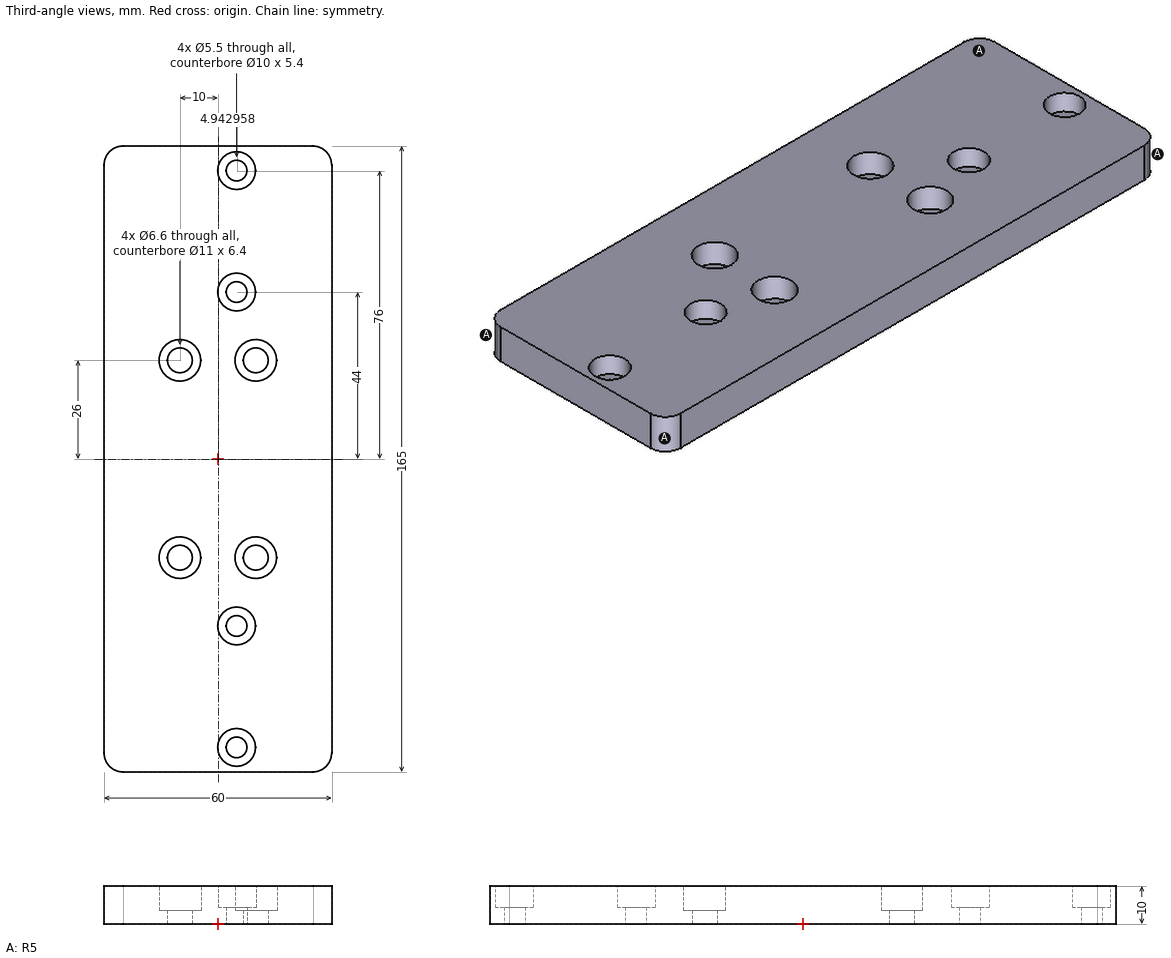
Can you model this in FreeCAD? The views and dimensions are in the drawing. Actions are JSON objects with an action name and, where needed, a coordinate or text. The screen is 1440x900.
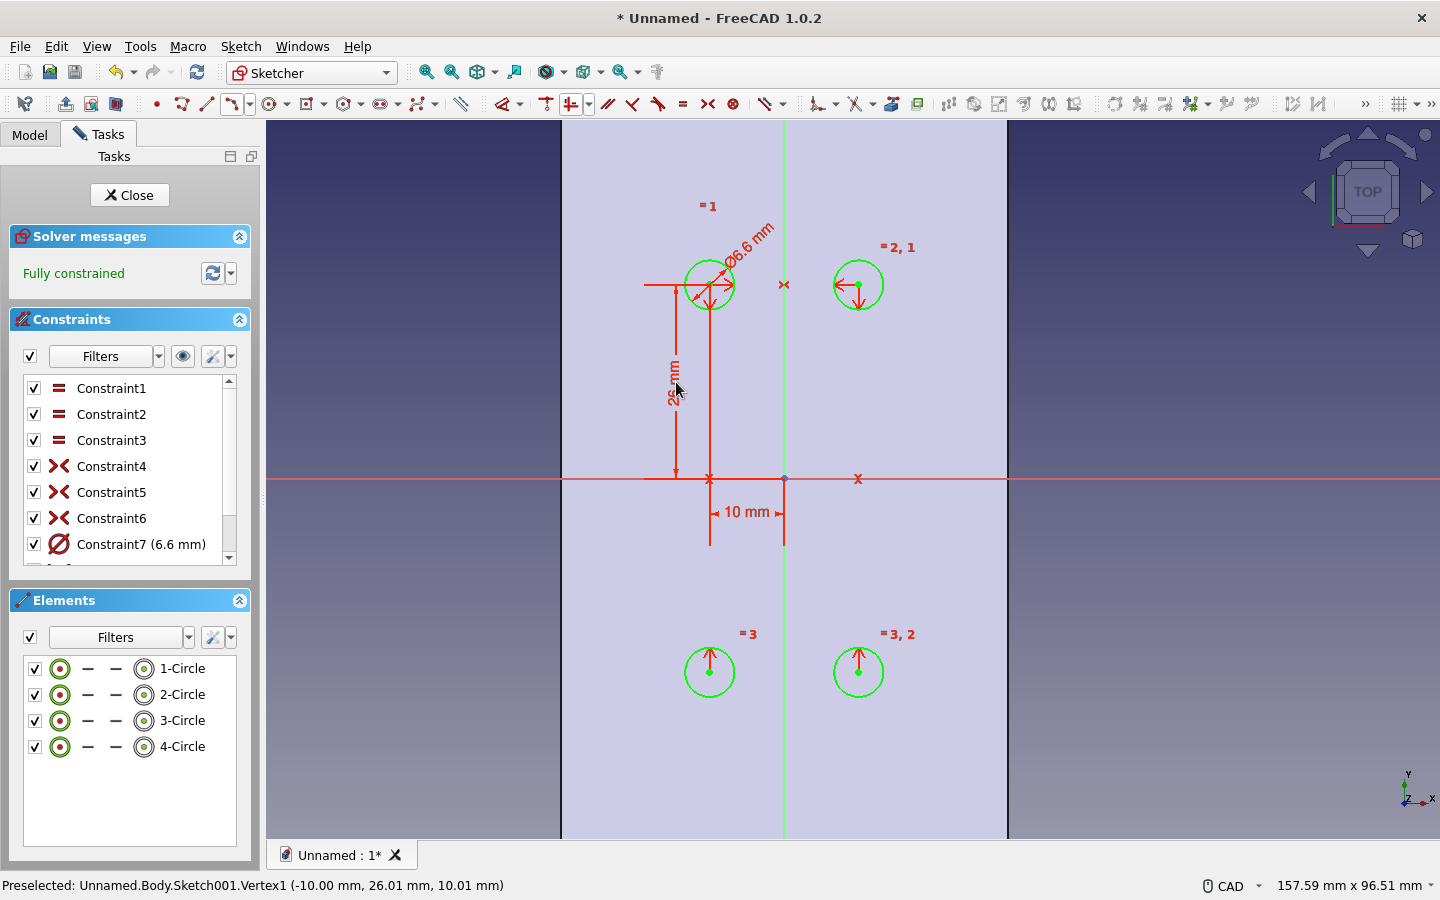
{"action": "left_click", "coordinate": [130, 195]}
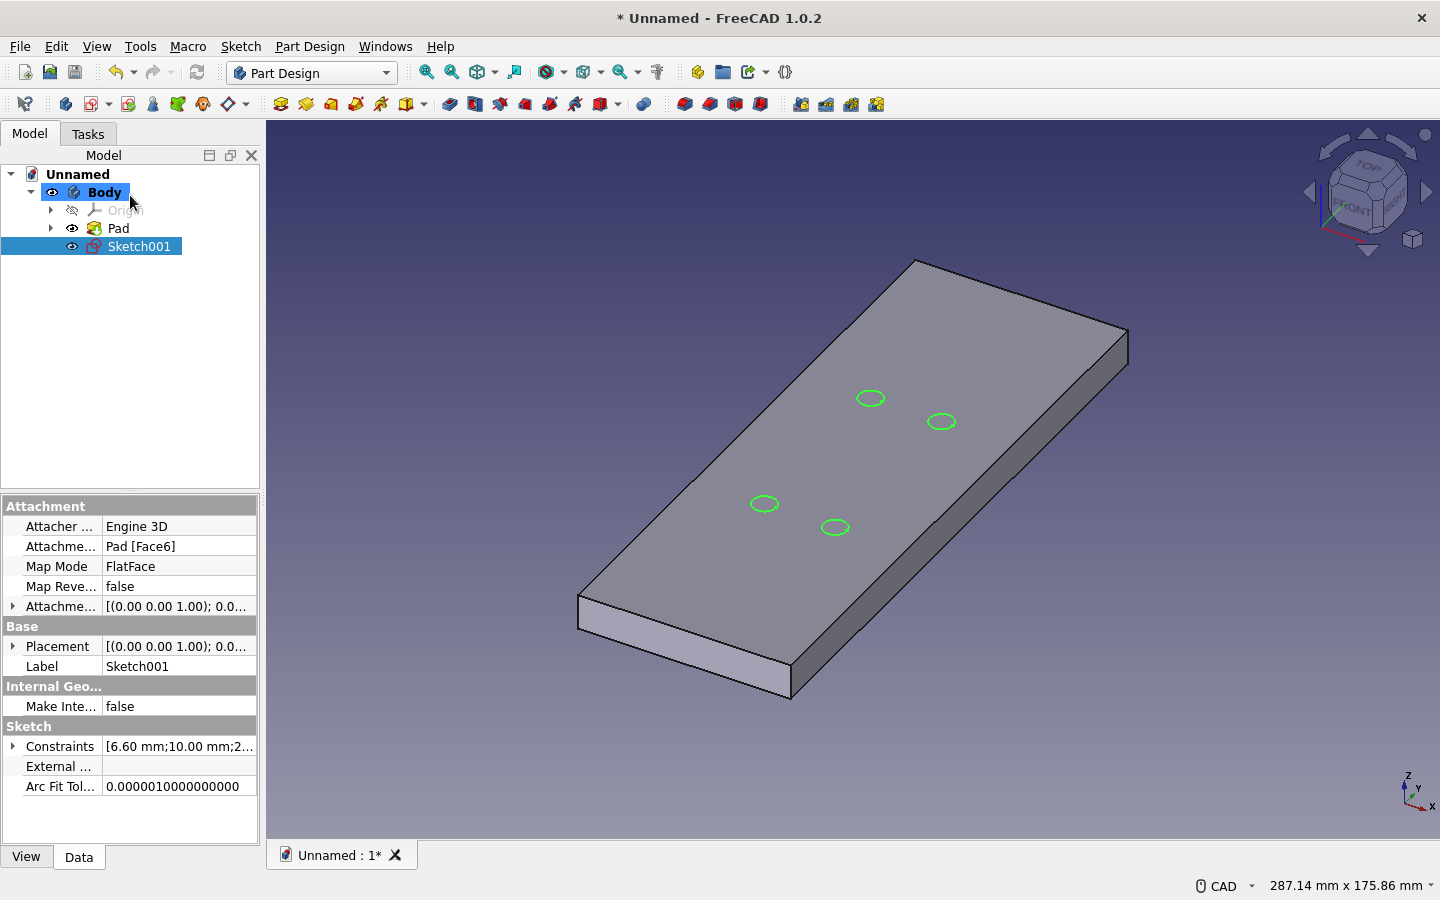
{"action": "left_click", "coordinate": [475, 104]}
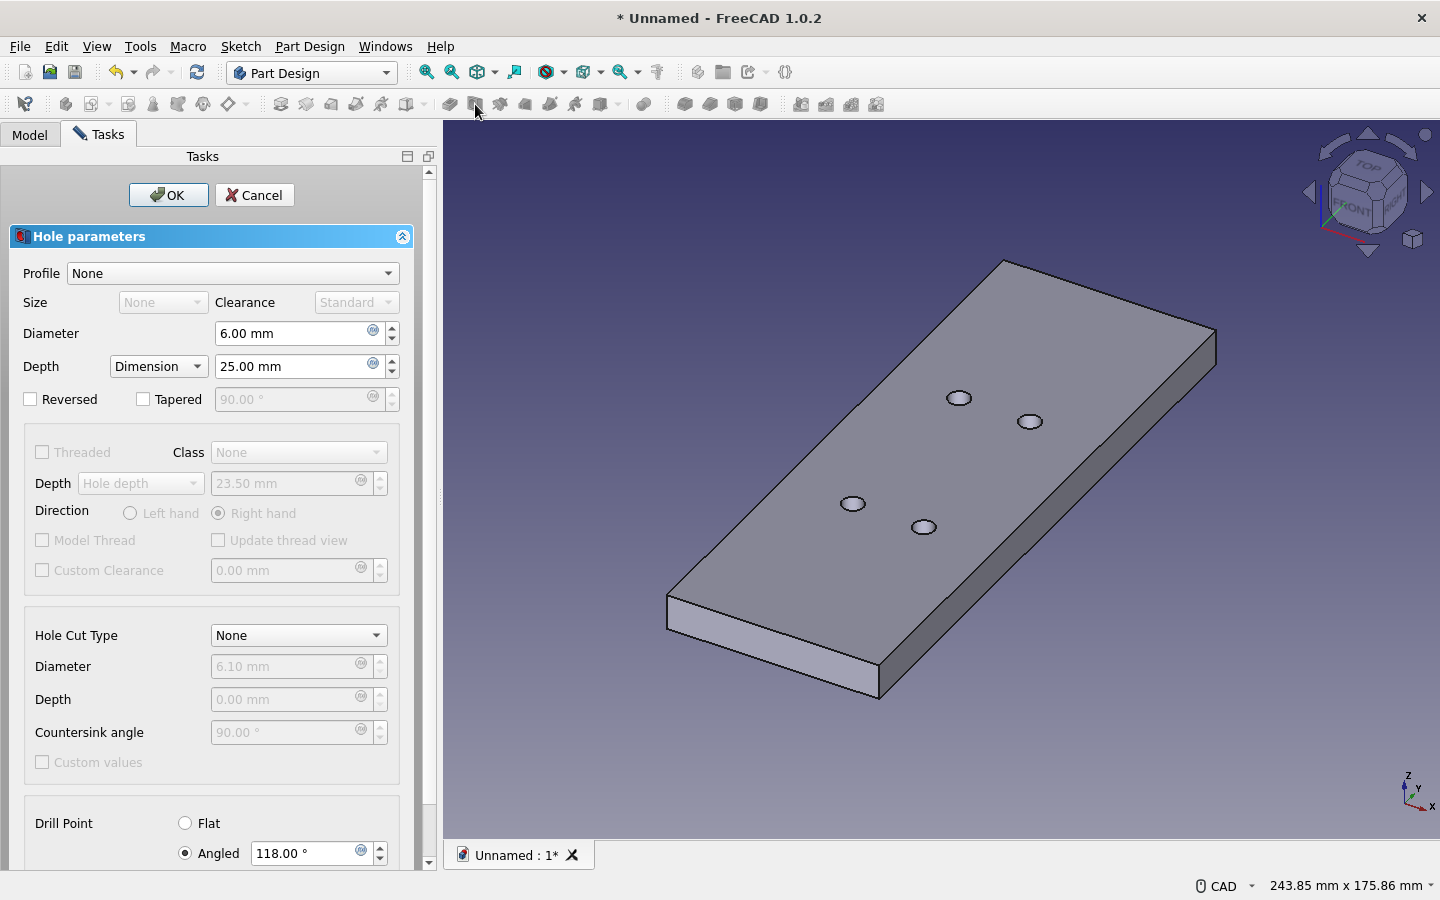
{"action": "triple_click", "coordinate": [300, 334]}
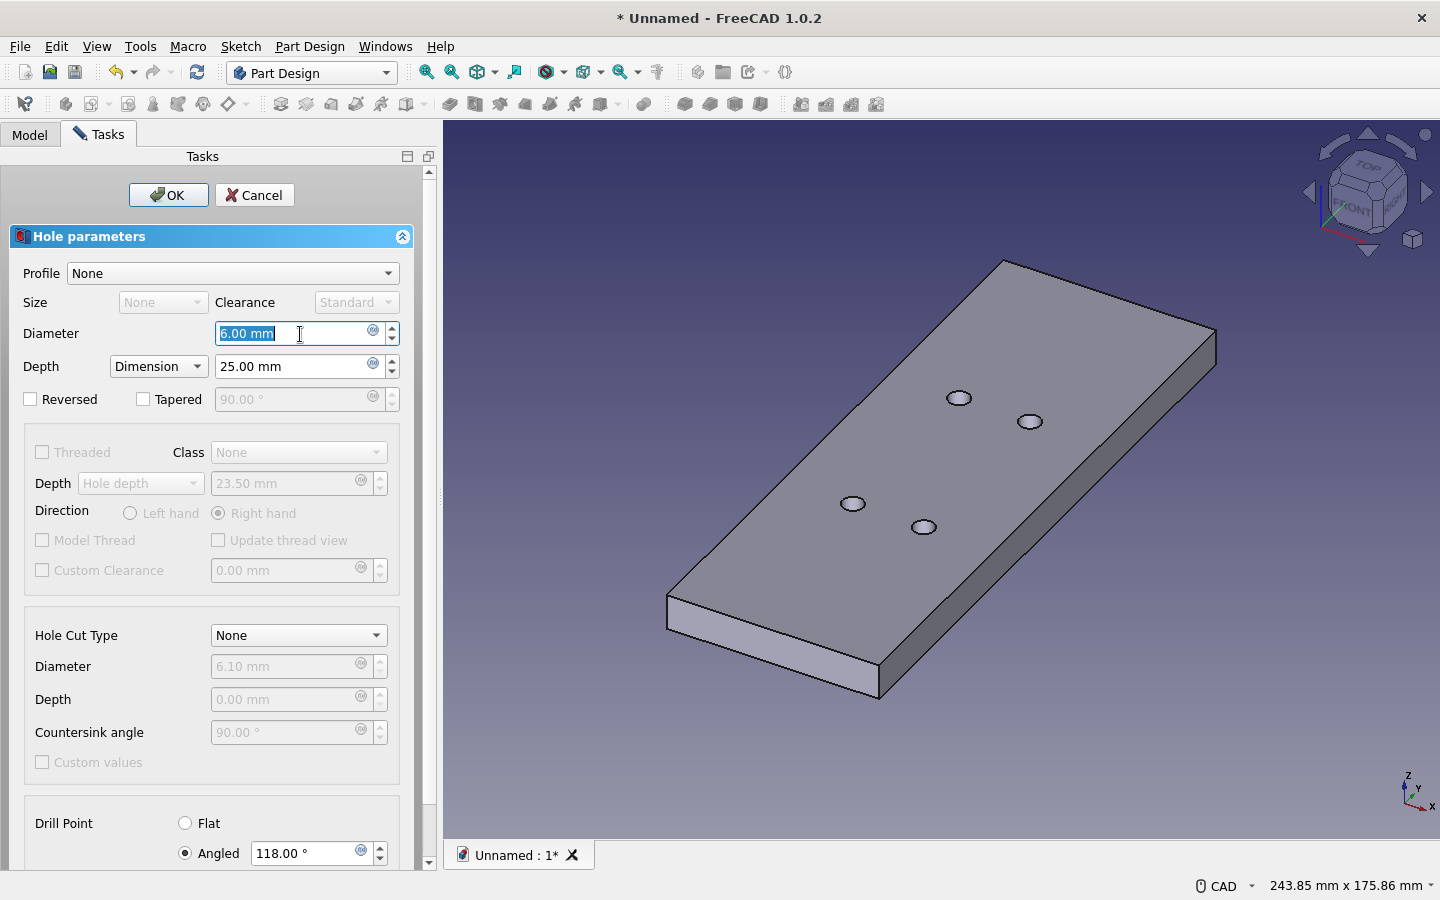
{"action": "type", "text": "6.6"}
{"action": "key", "text": "Tab"}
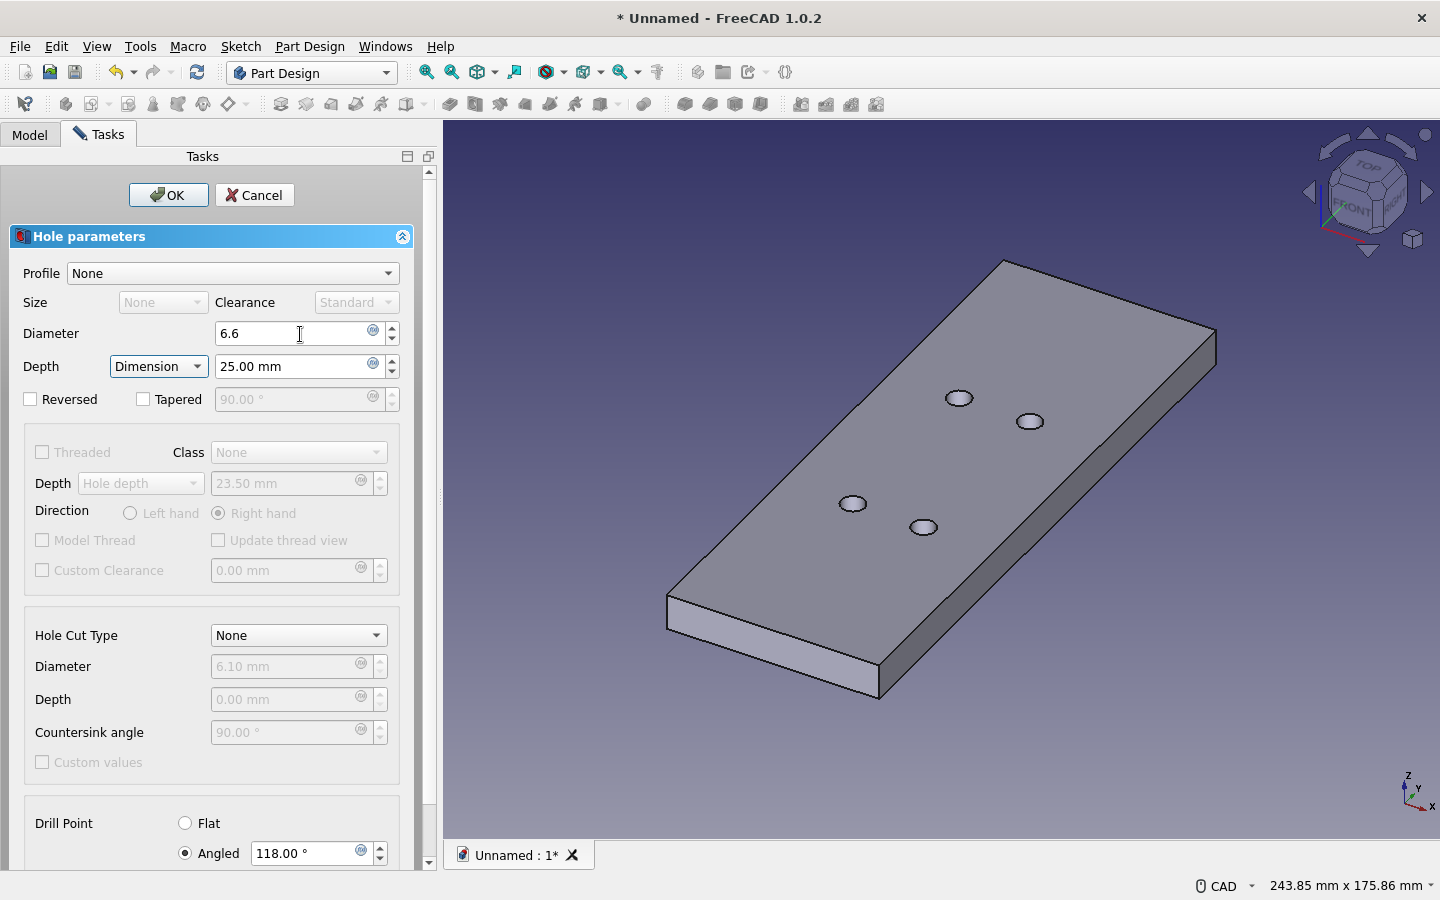
{"action": "left_click", "coordinate": [160, 366]}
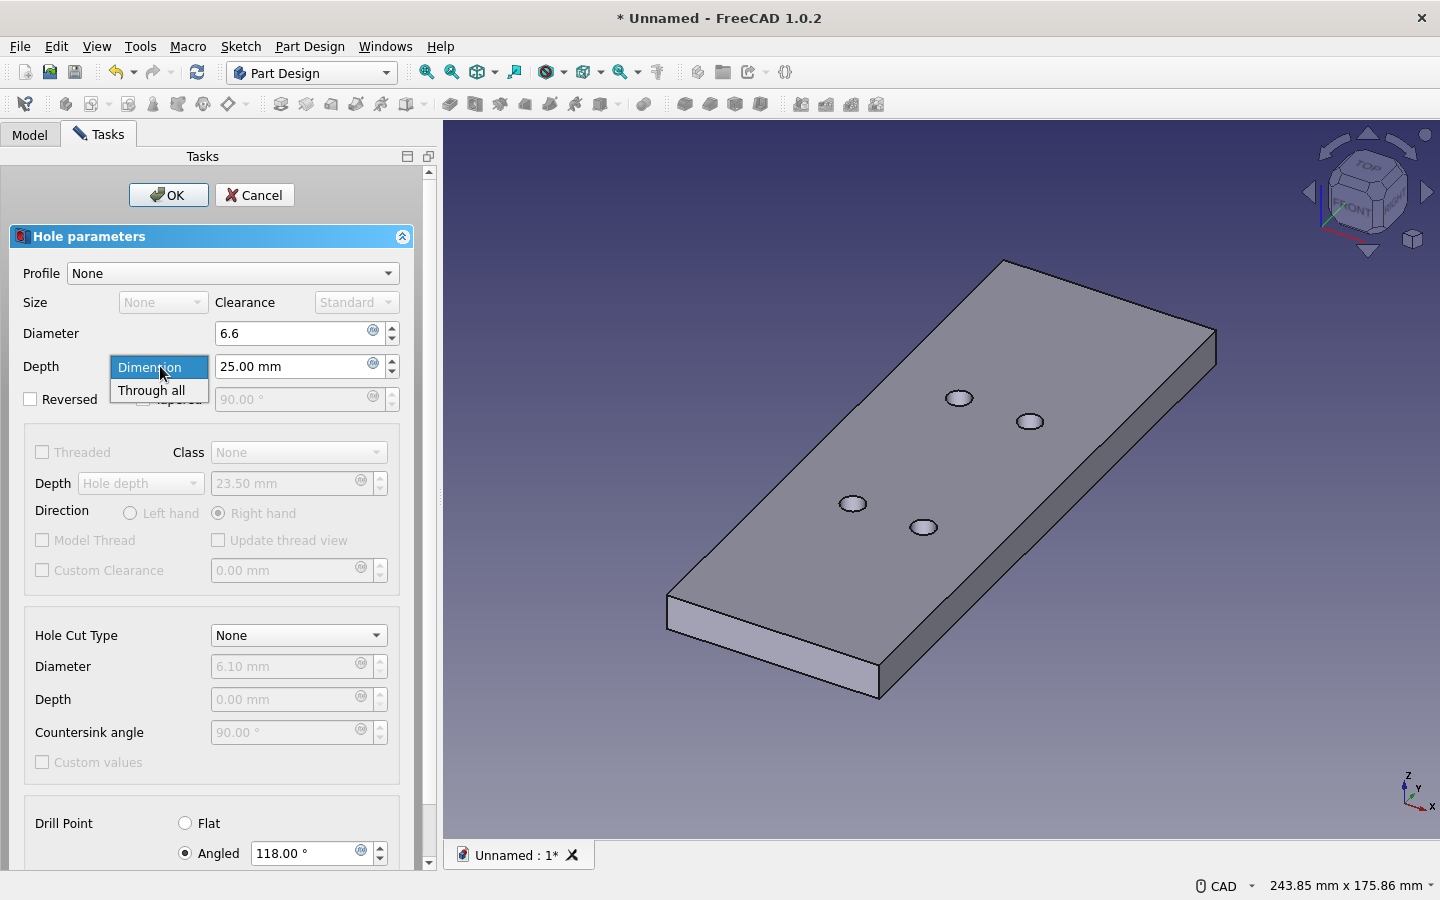
{"action": "left_click", "coordinate": [158, 390]}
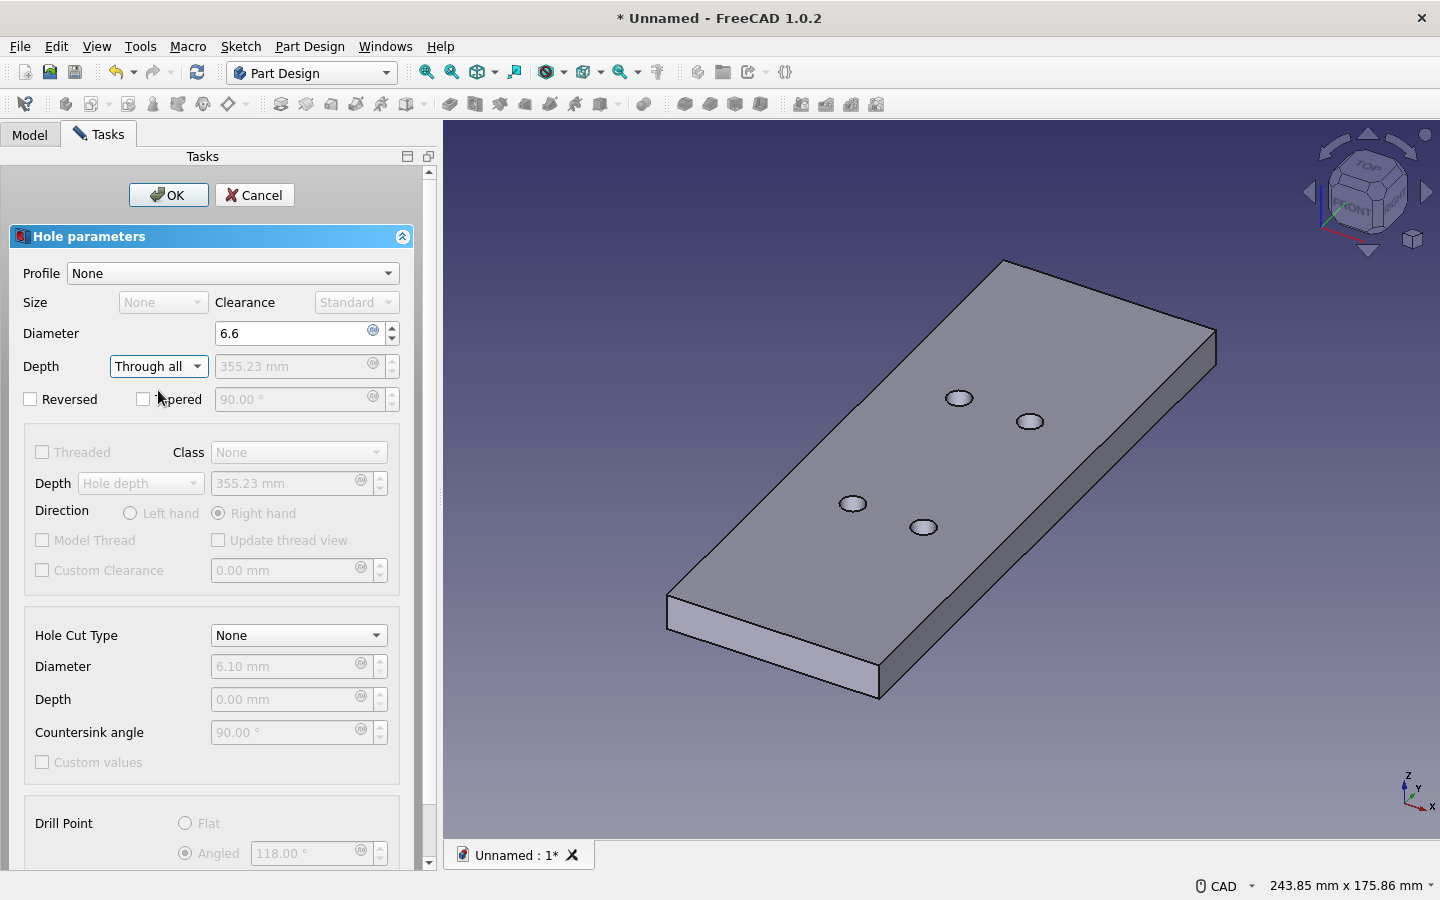
{"action": "left_click", "coordinate": [300, 636]}